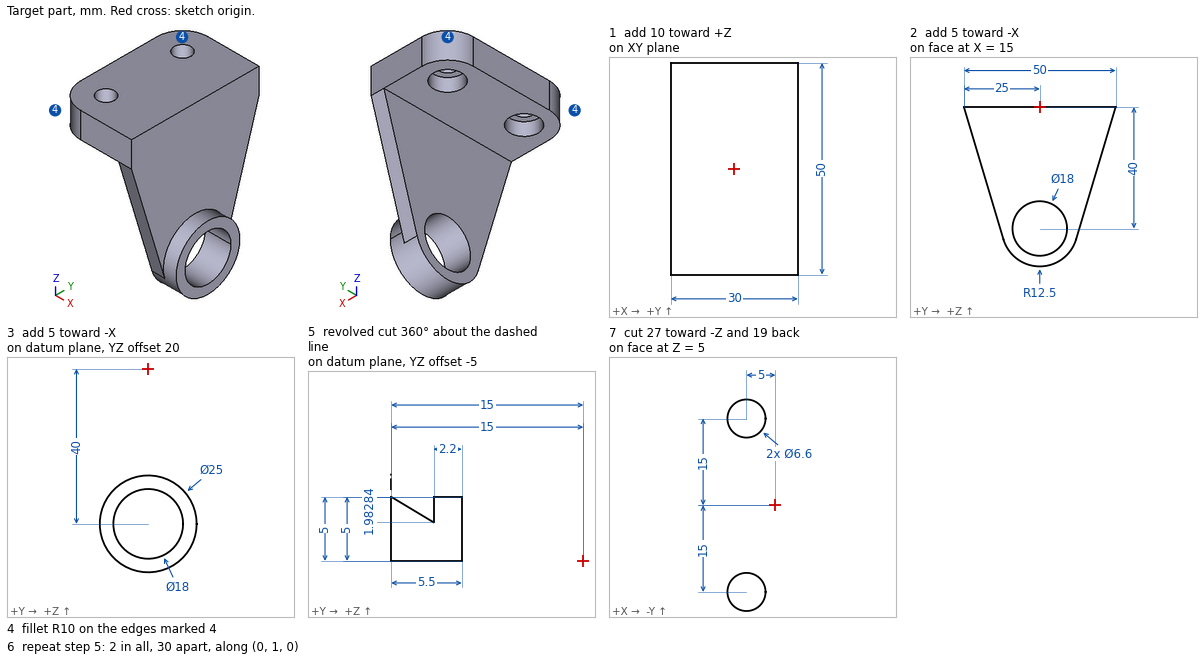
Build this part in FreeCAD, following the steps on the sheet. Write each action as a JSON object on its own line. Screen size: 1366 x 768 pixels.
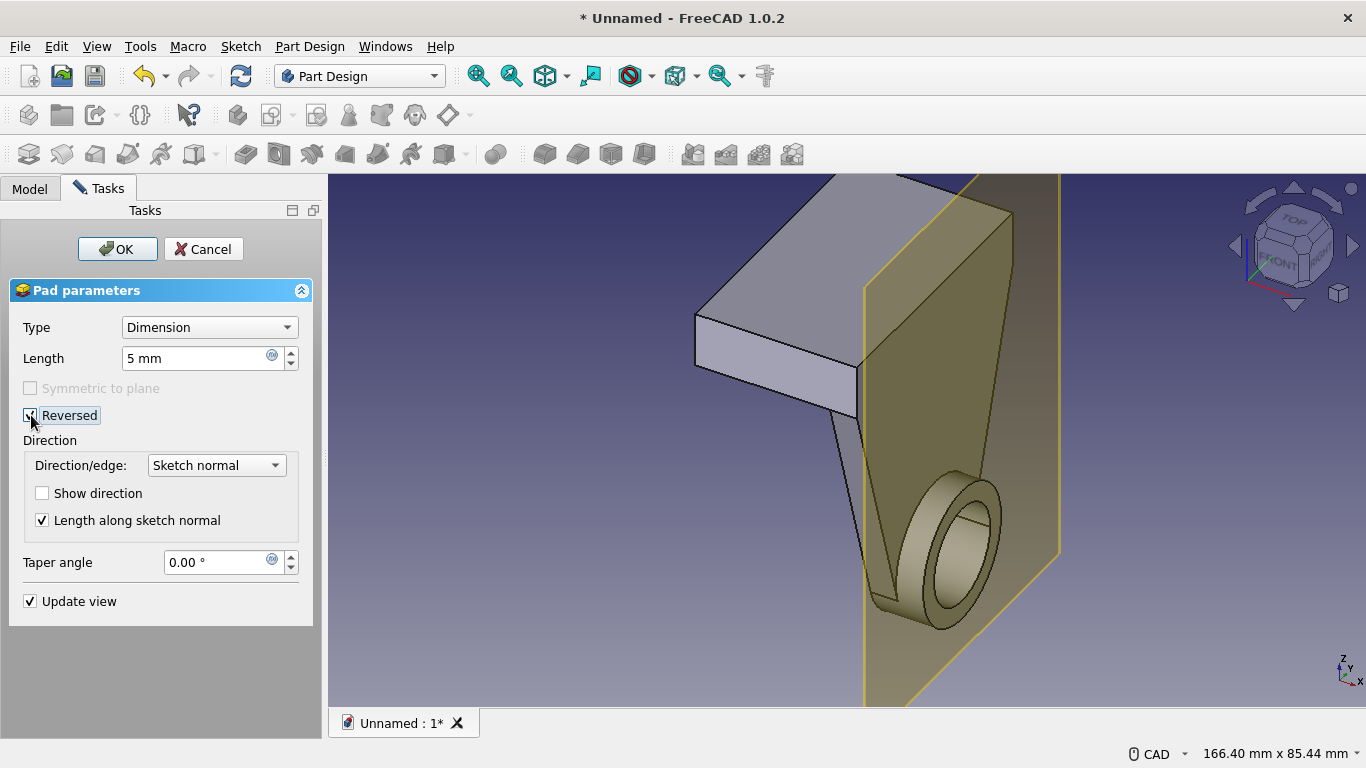
{"action": "left_click", "coordinate": [118, 249]}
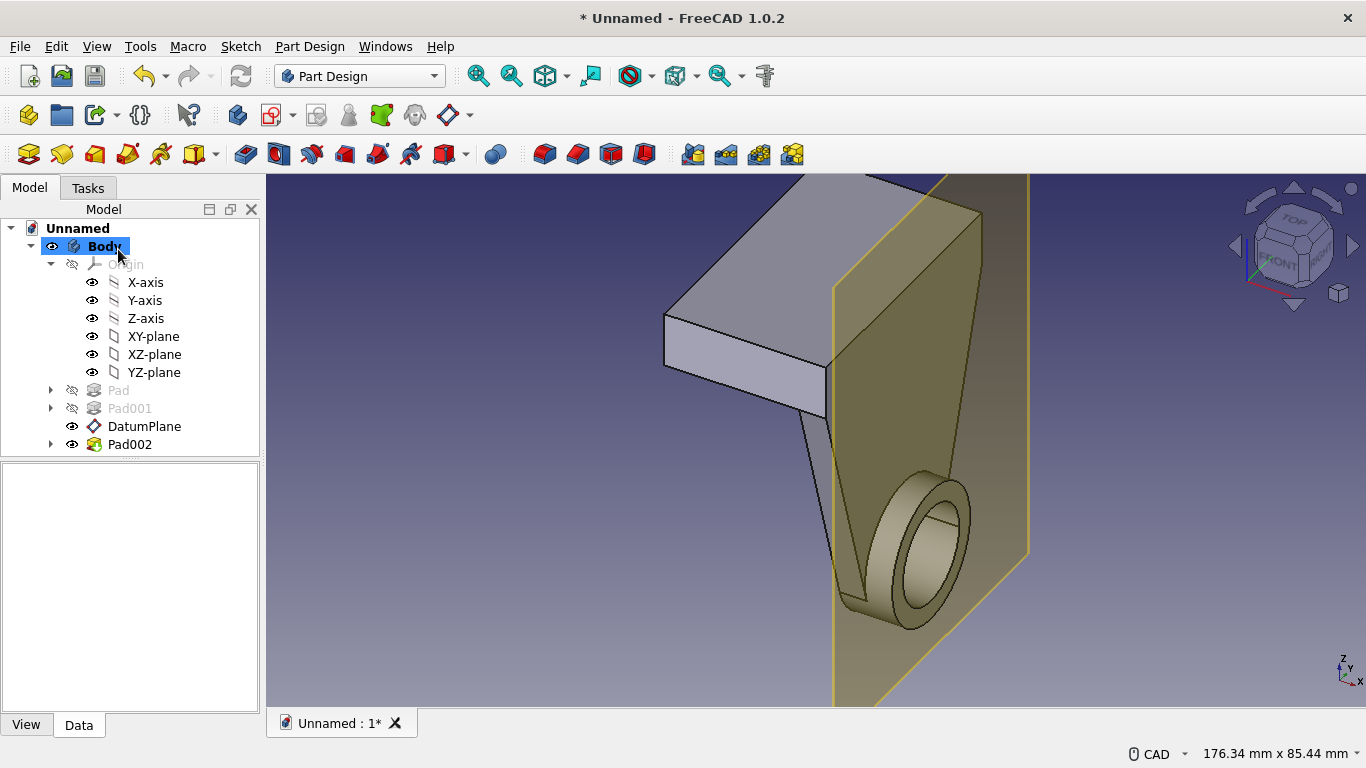
{"action": "left_click", "coordinate": [117, 426]}
{"action": "key", "text": "space"}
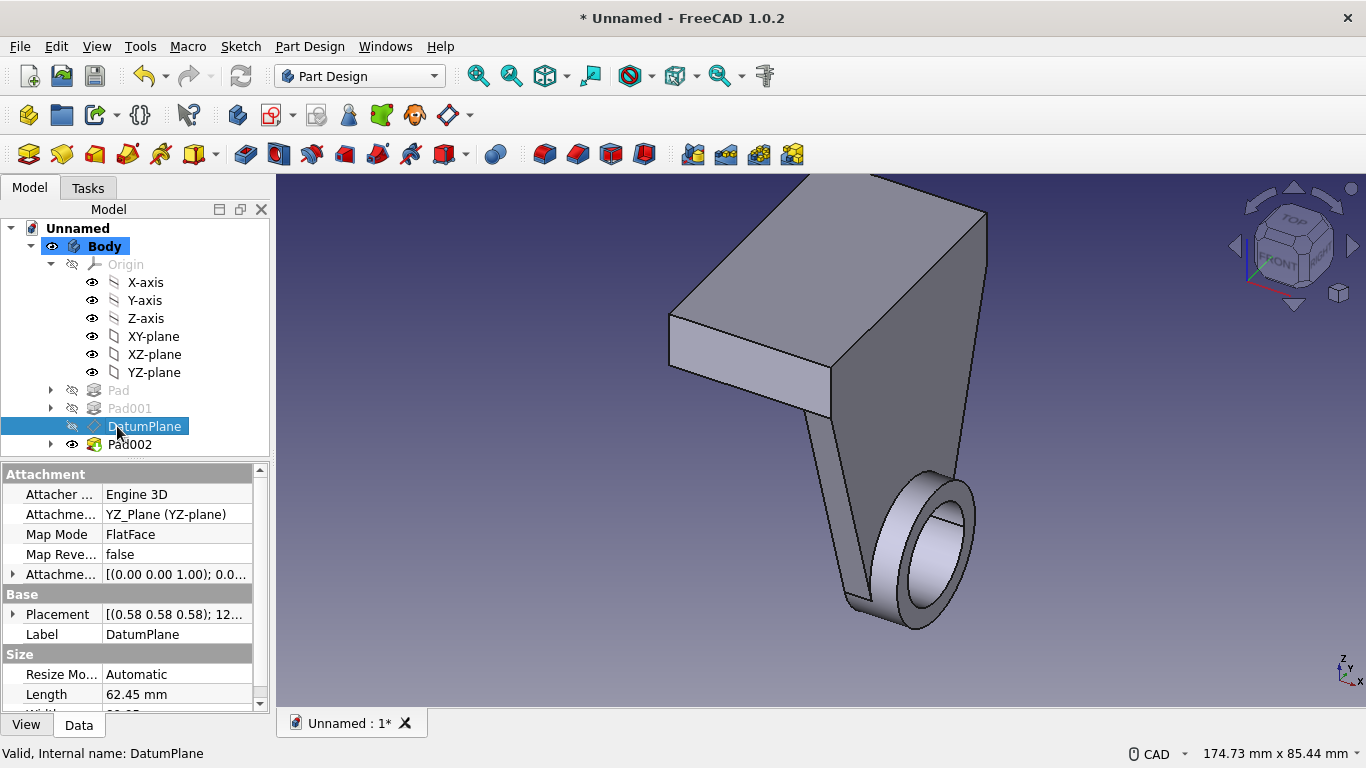
{"action": "key", "text": "v f"}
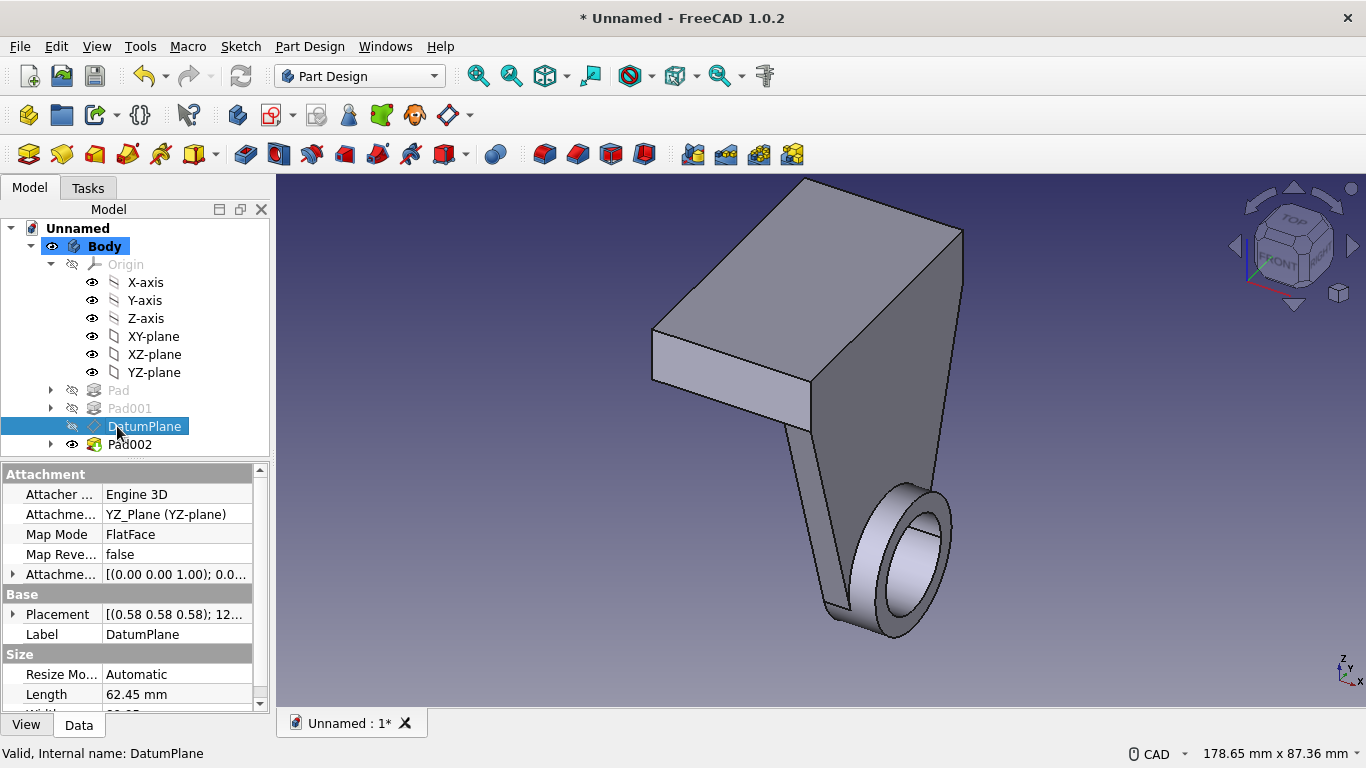
{"action": "key", "text": "0"}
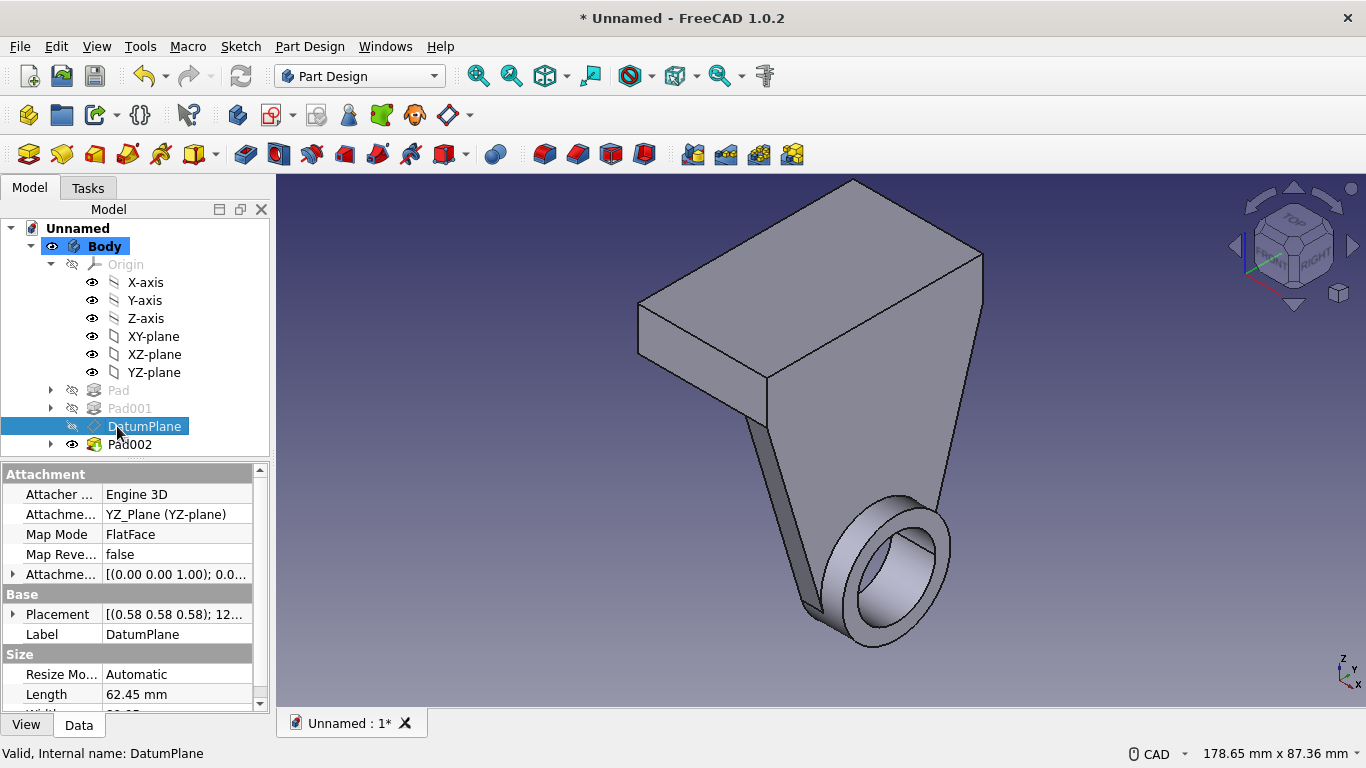
{"action": "key", "text": "2"}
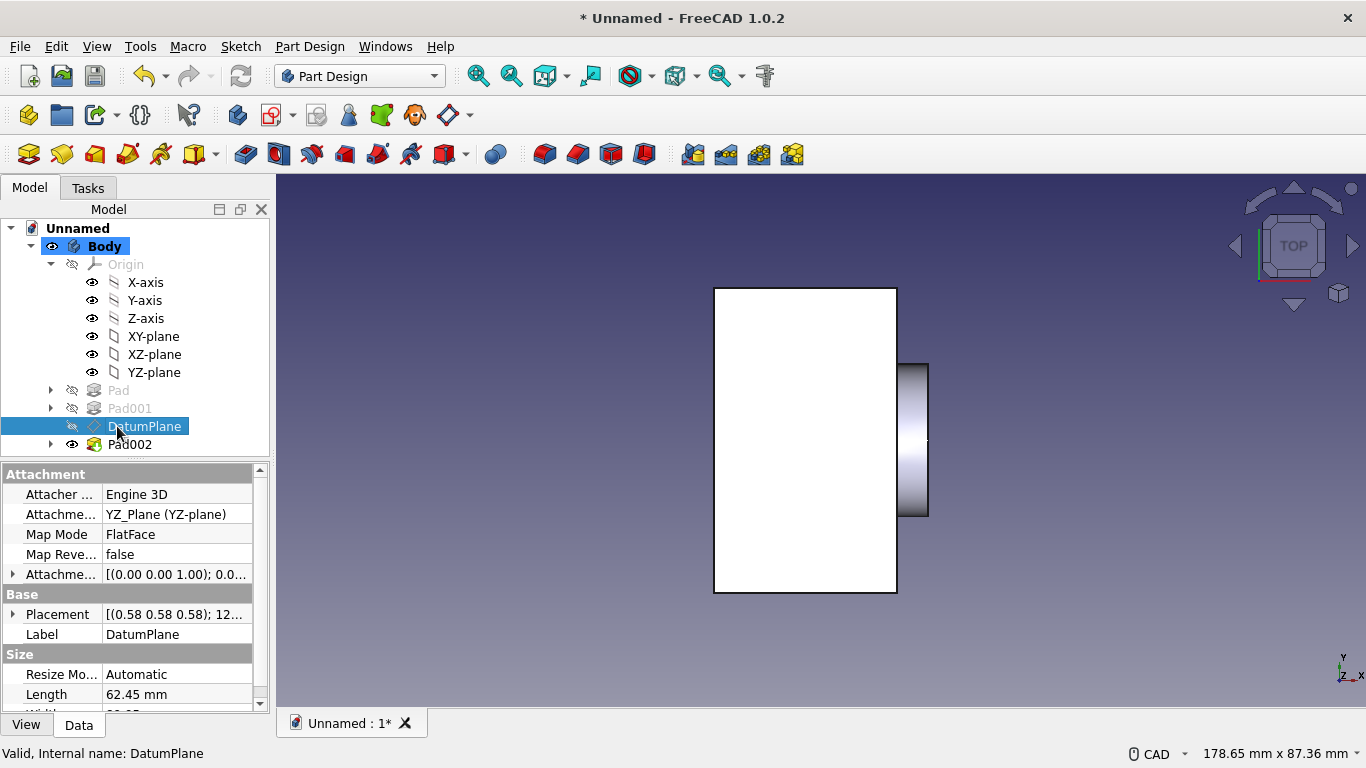
{"action": "key", "text": "1"}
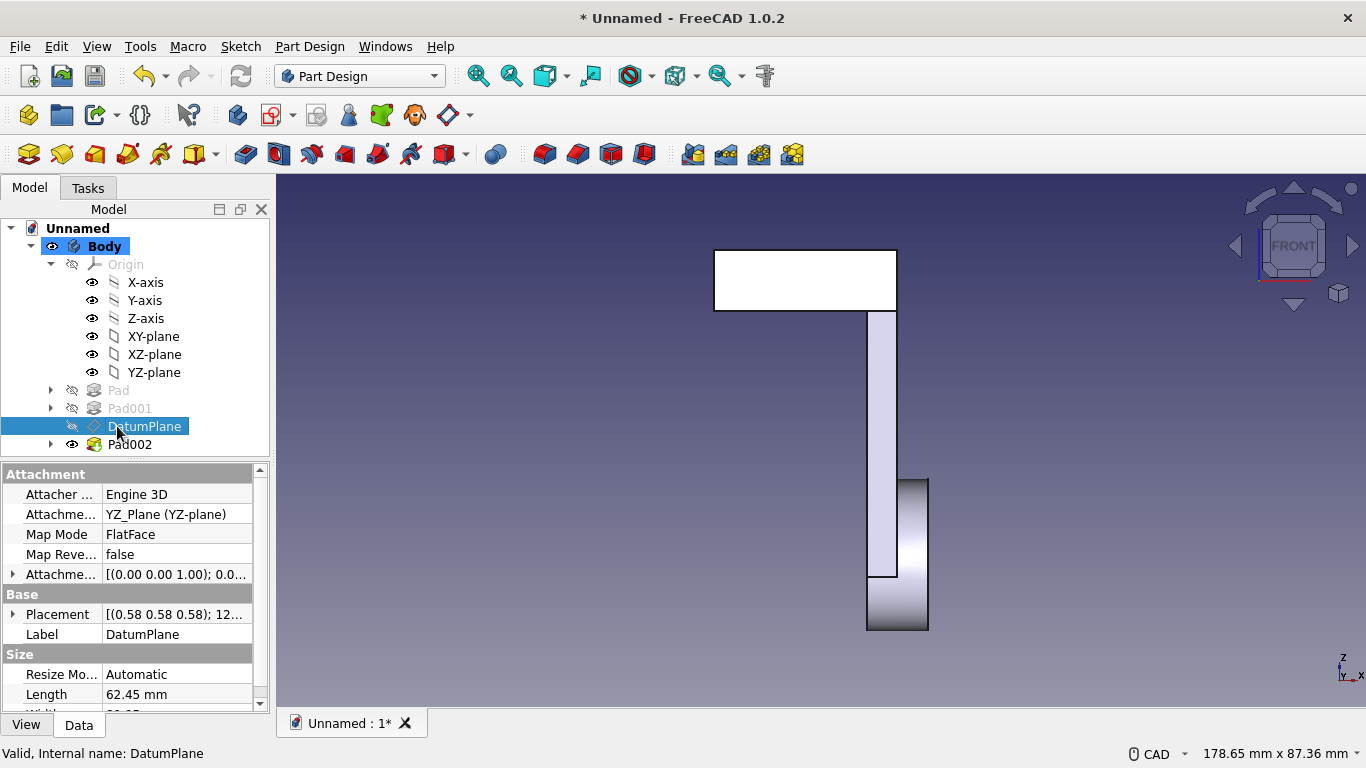
{"action": "left_click", "coordinate": [714, 279]}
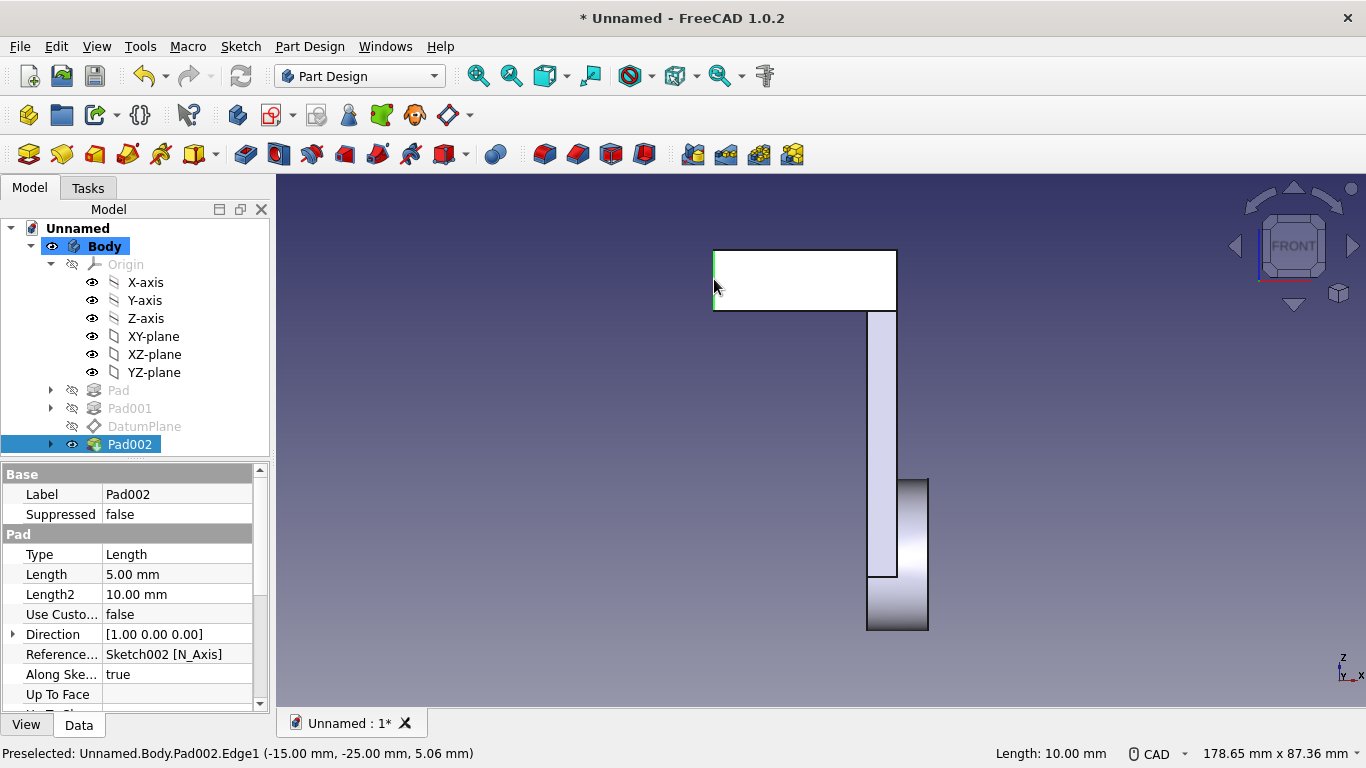
{"action": "key", "text": "3"}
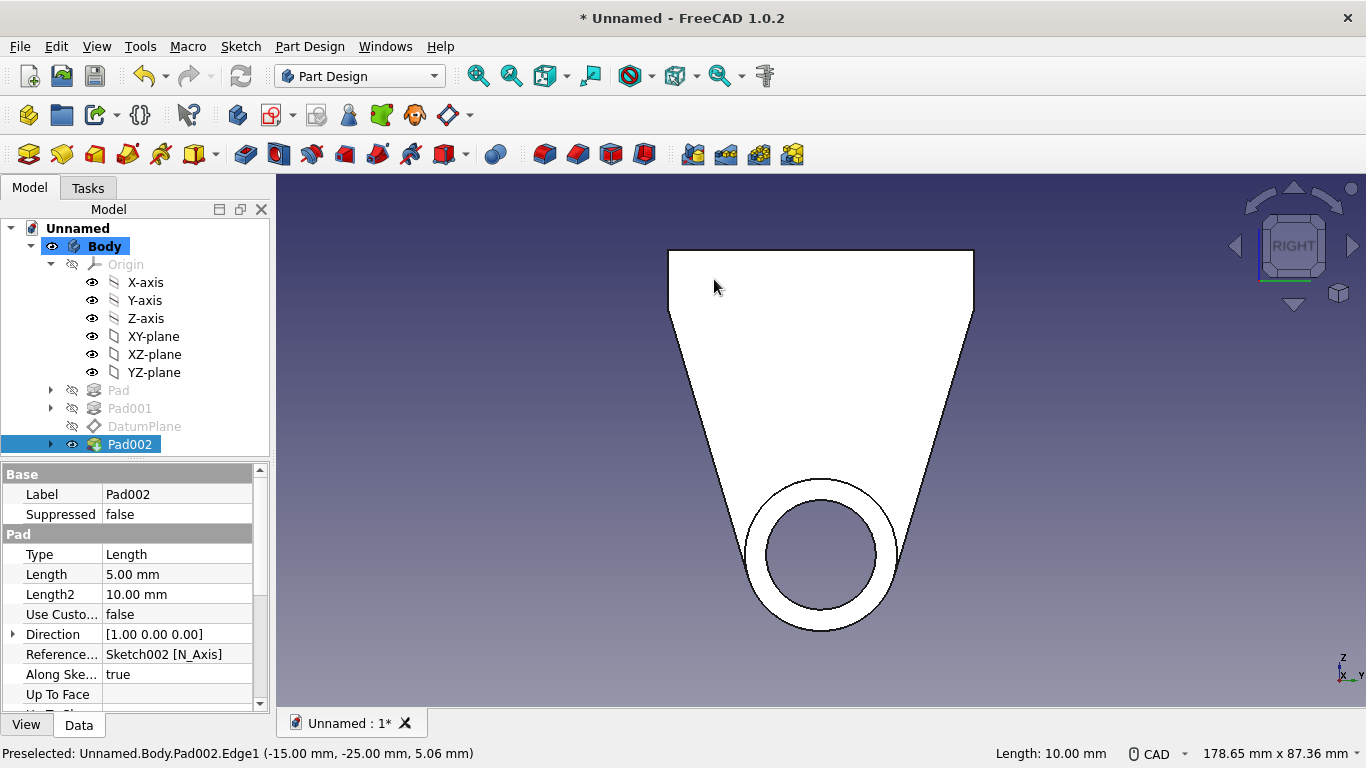
{"action": "key", "text": "5"}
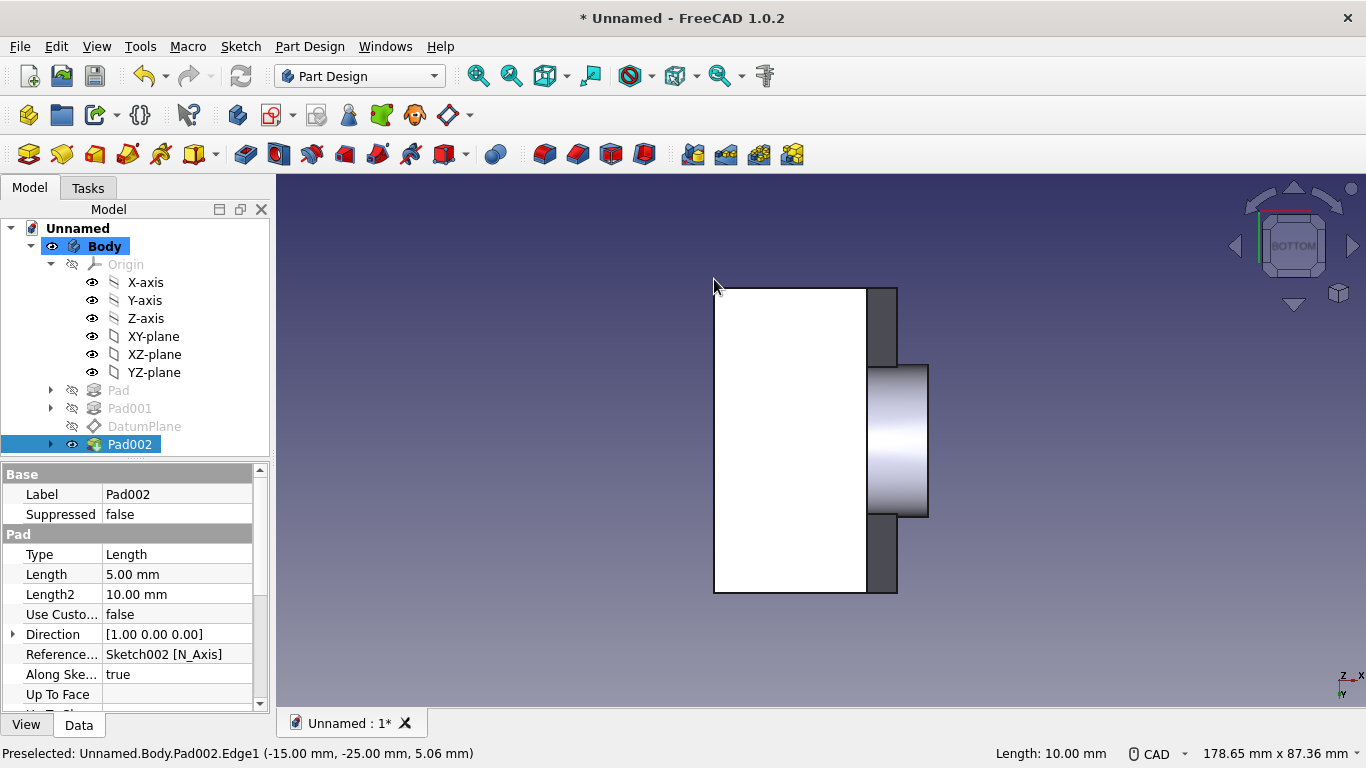
{"action": "key", "text": "4"}